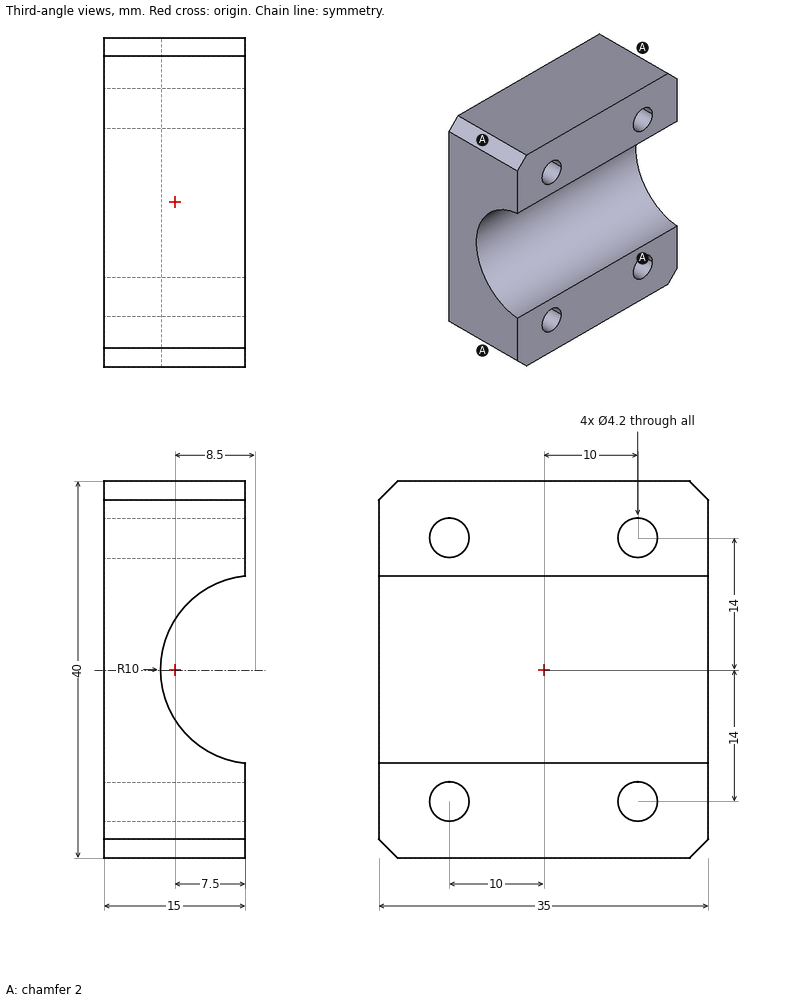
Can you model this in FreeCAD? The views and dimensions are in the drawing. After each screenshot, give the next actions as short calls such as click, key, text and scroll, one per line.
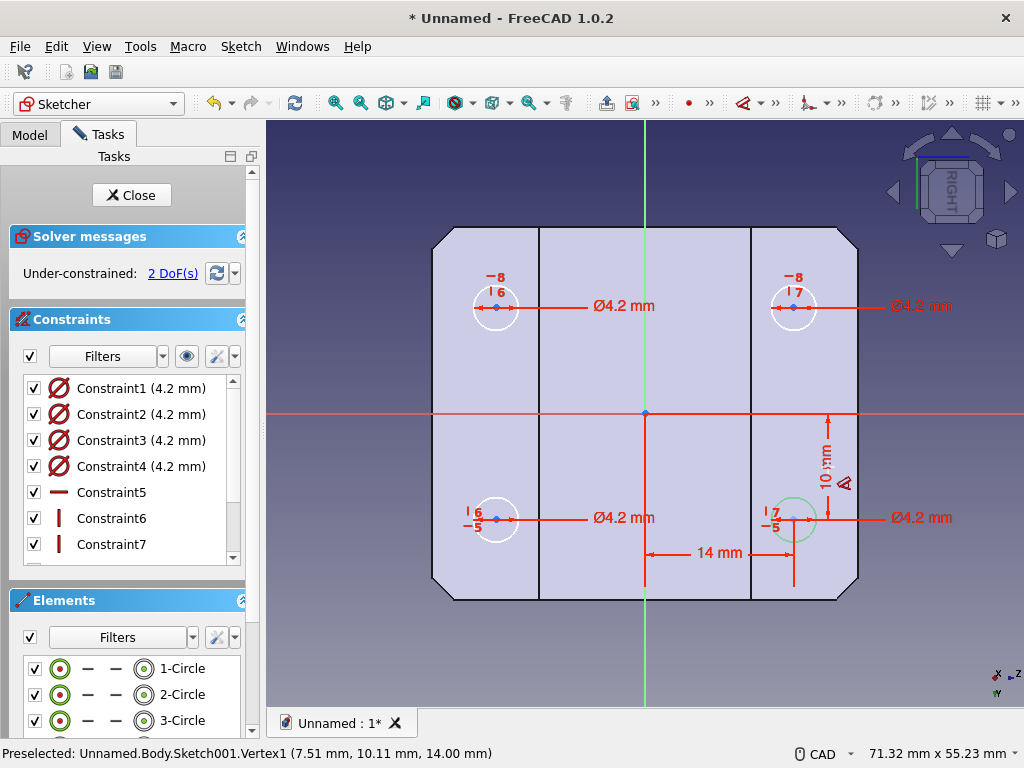
click(496, 520)
click(571, 554)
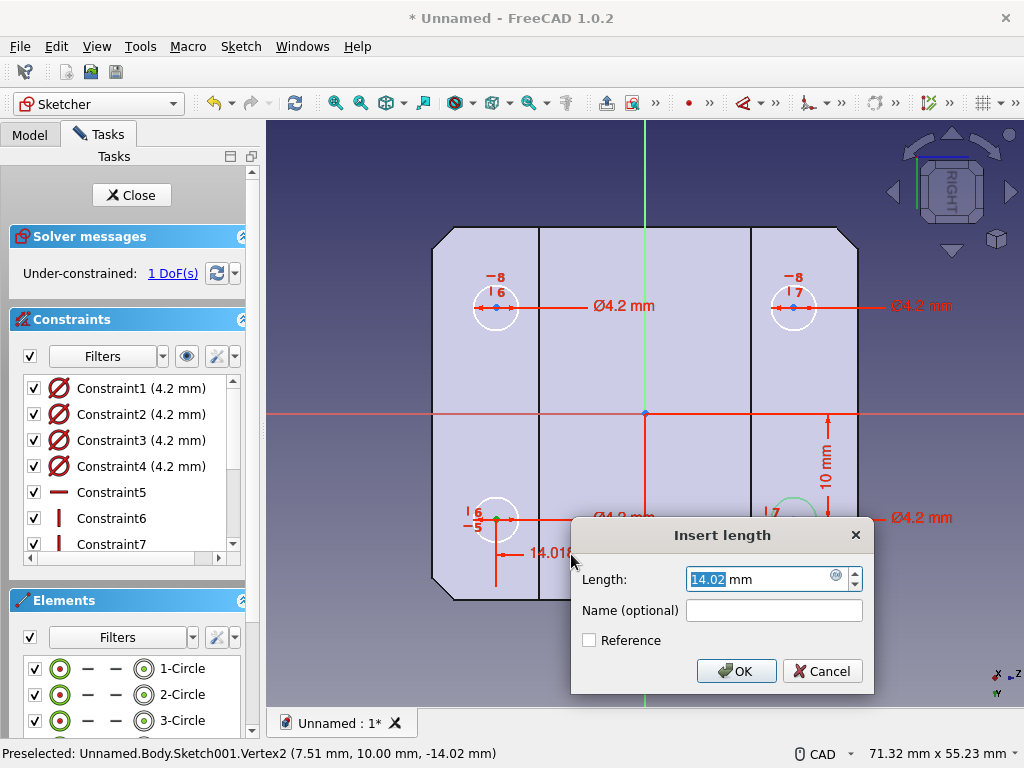
text(14)
key(Return)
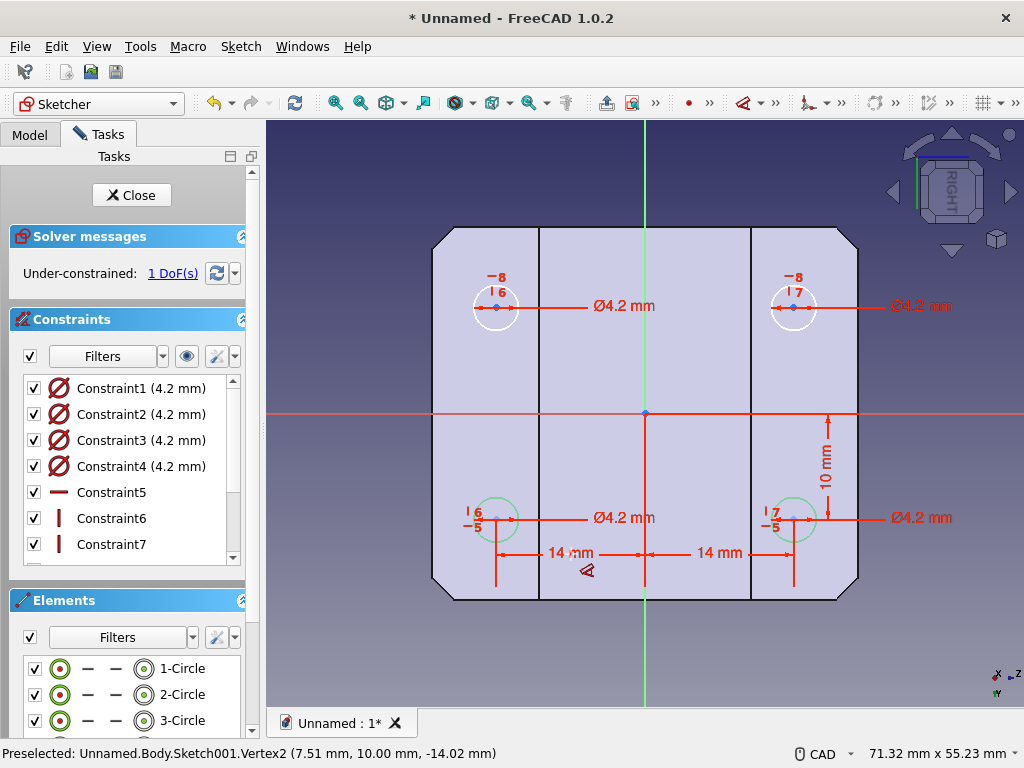
click(496, 308)
click(462, 361)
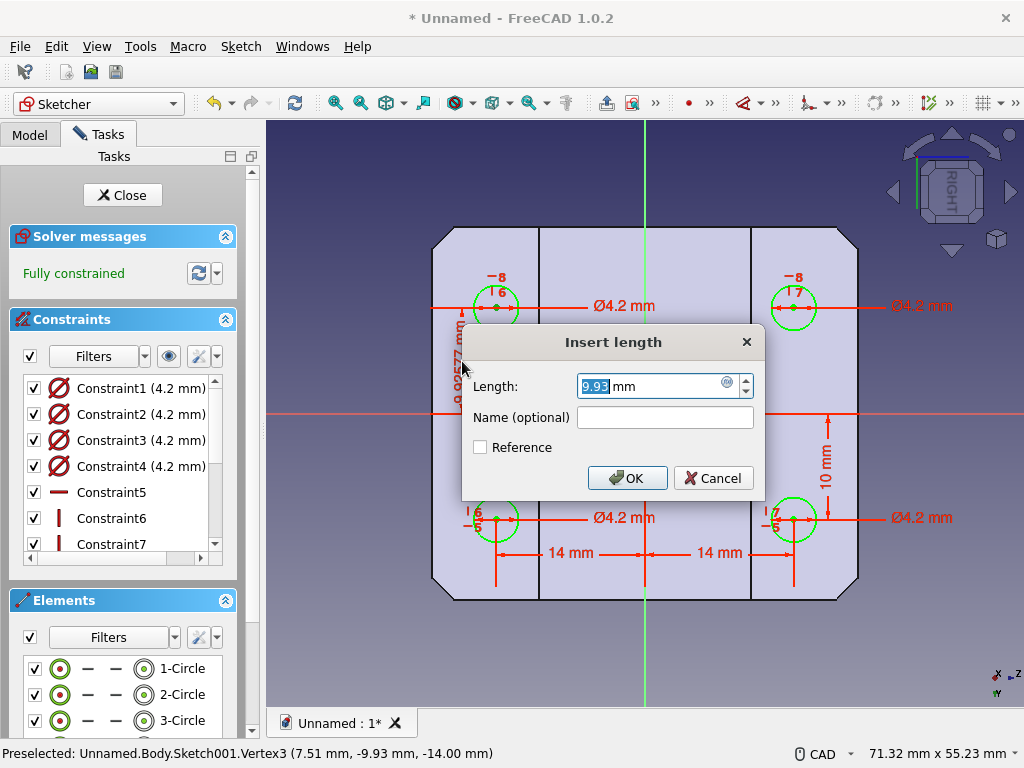
text(10)
key(Return)
key(Escape)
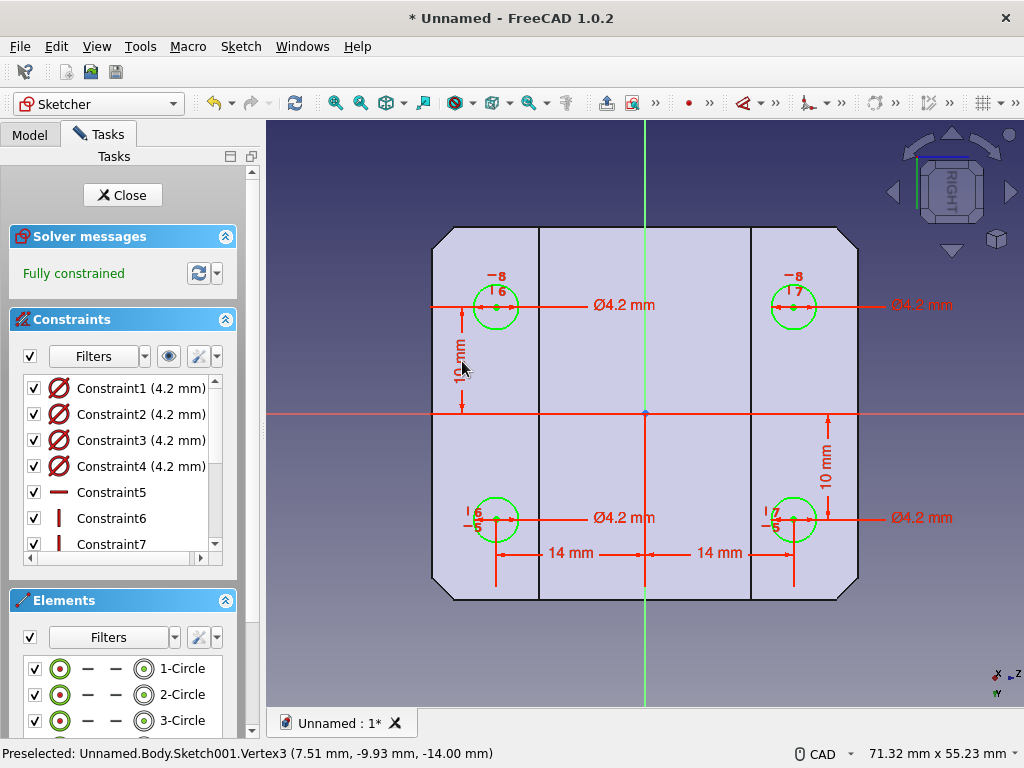
click(123, 195)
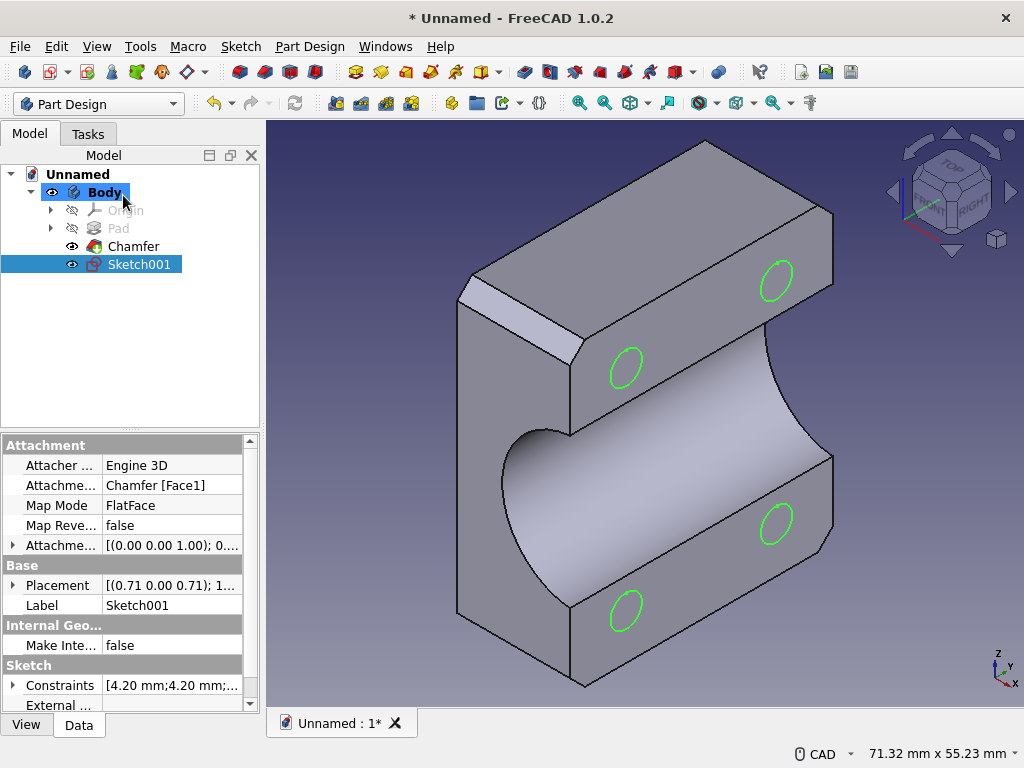
click(550, 72)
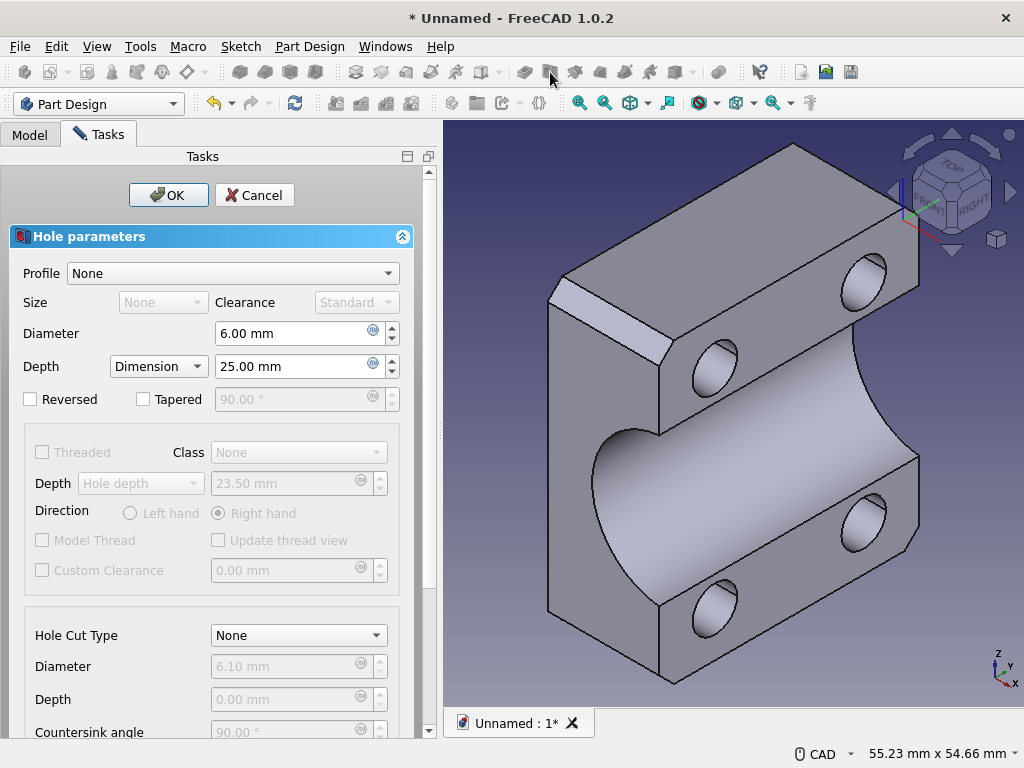
triple_click(300, 334)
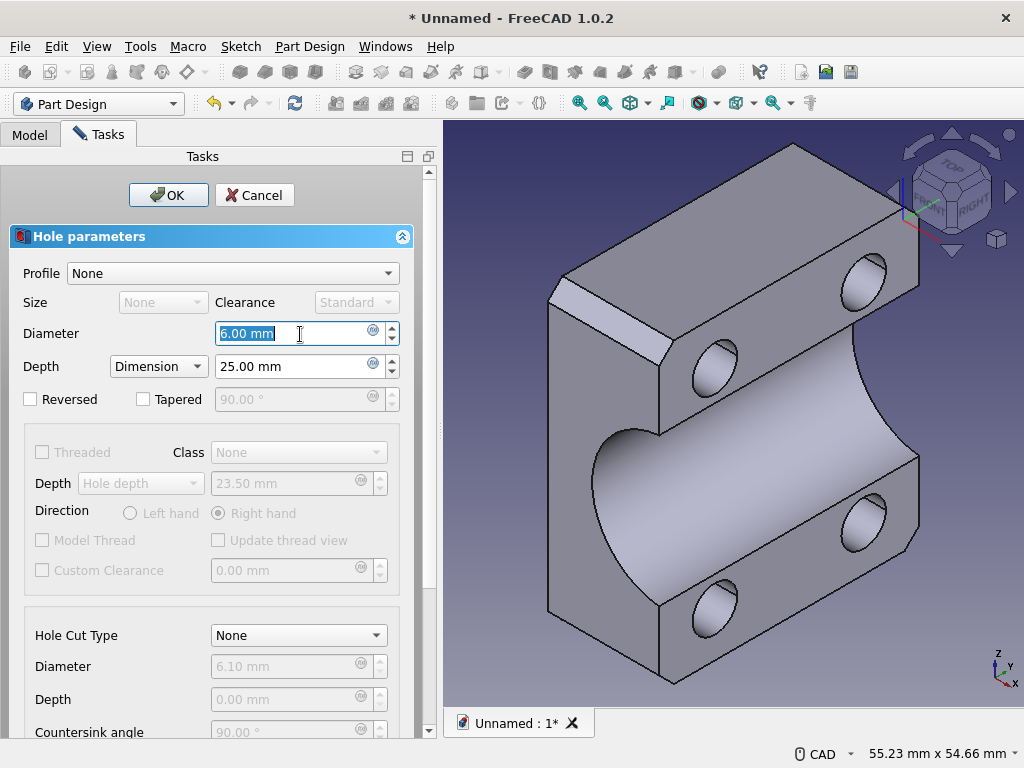
text(4.2)
key(Tab)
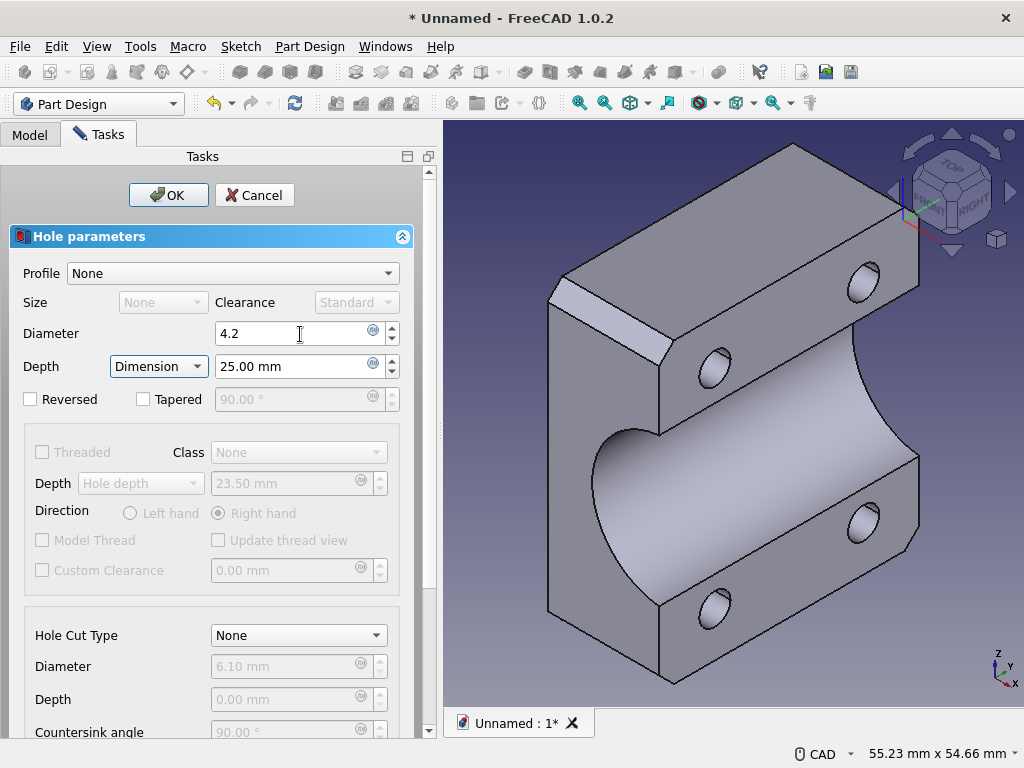
click(160, 366)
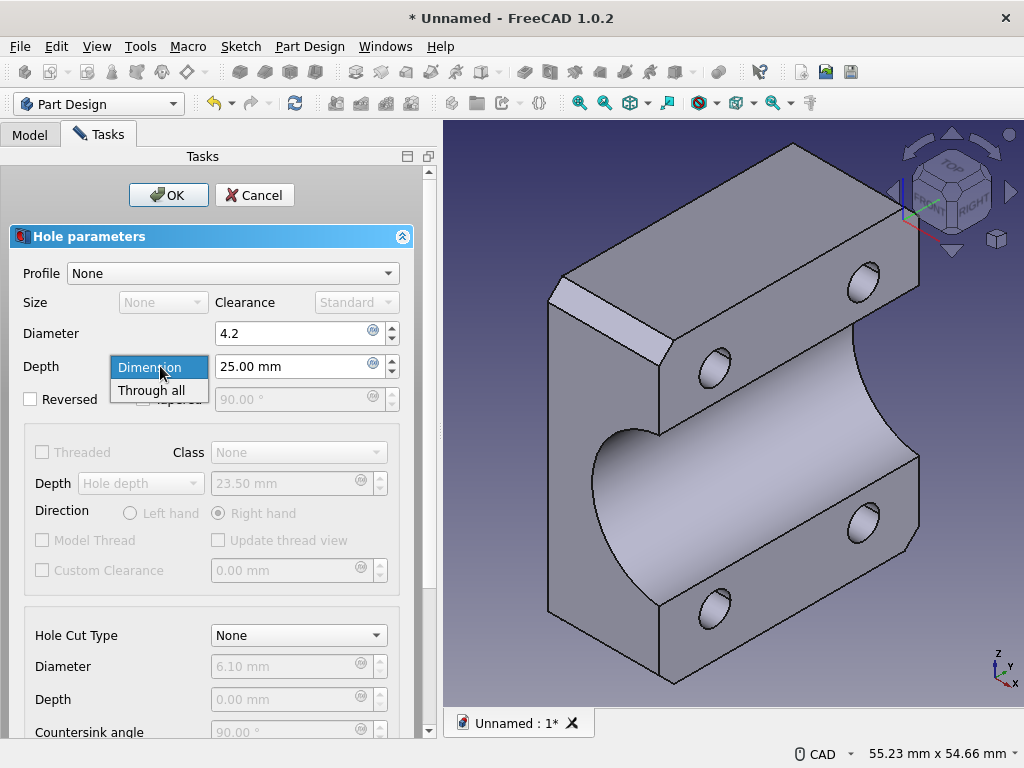
click(158, 390)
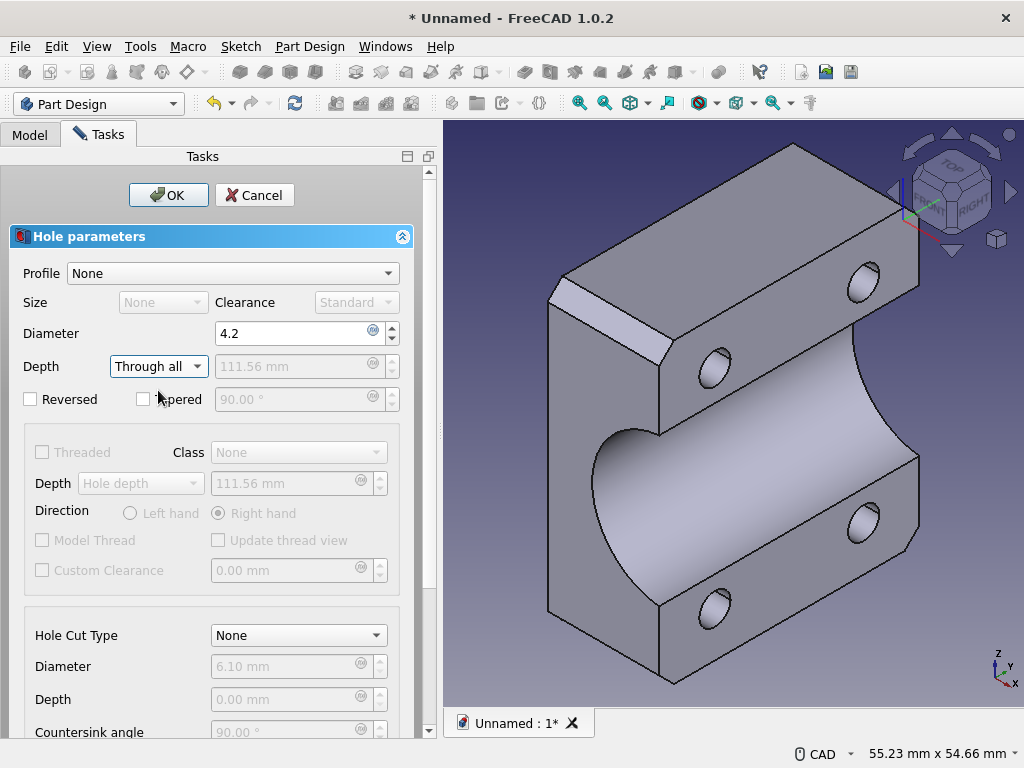
click(169, 195)